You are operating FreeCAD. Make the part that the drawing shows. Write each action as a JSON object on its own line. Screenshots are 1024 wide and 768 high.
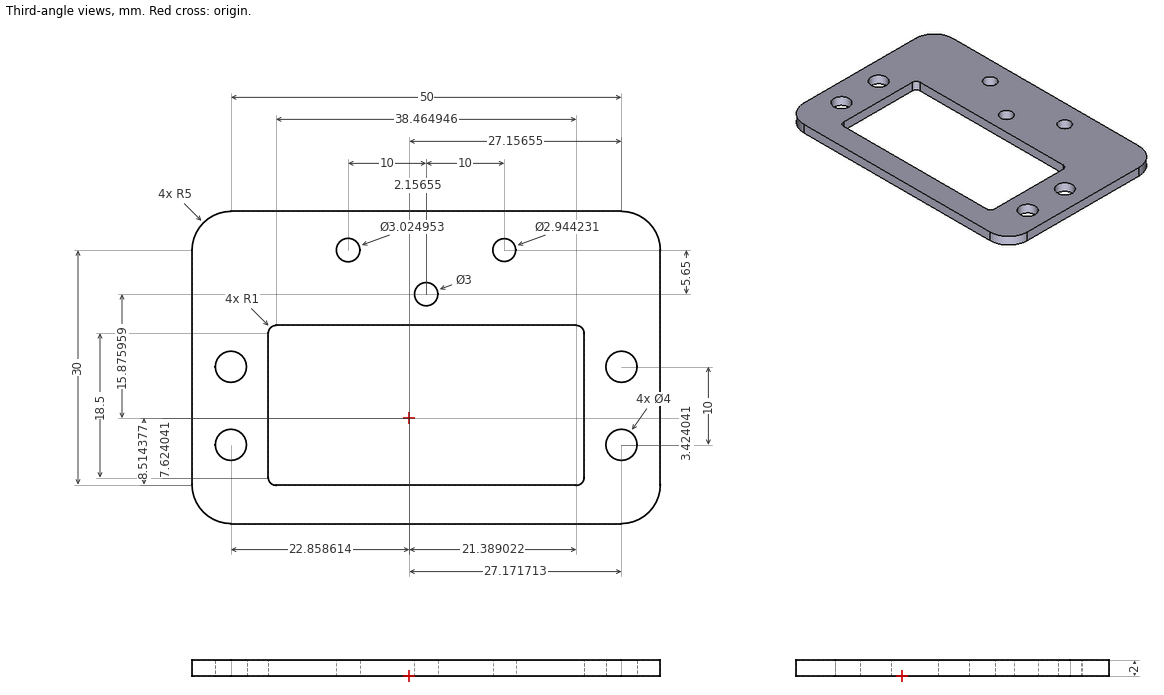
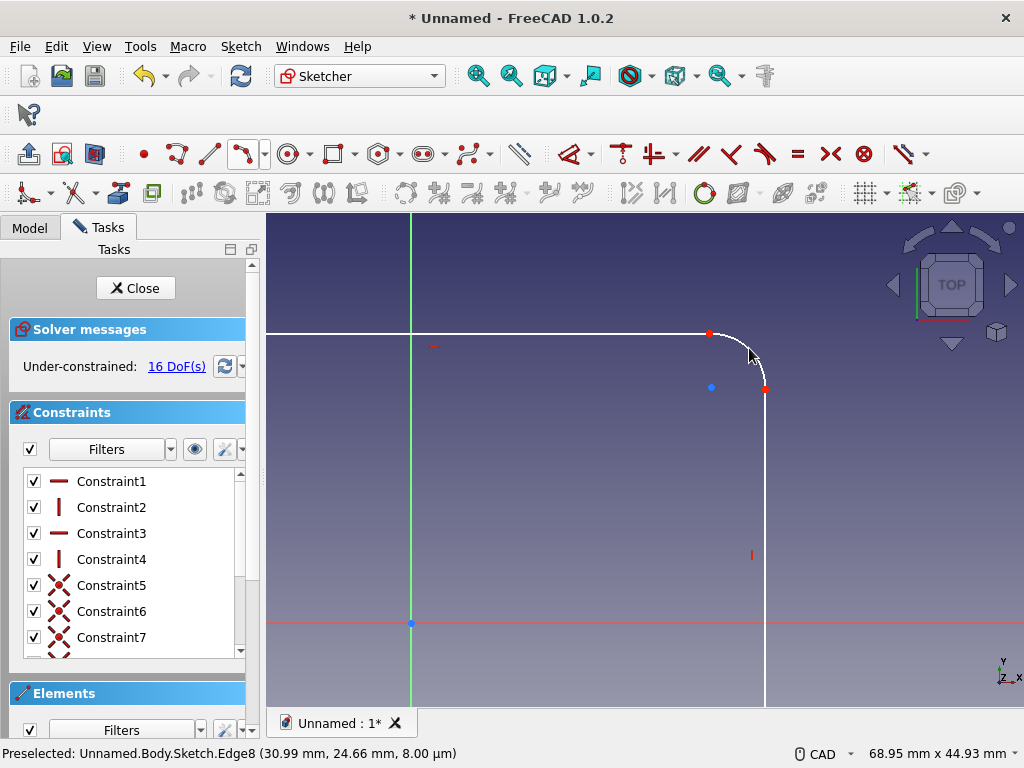
{"action": "left_click", "coordinate": [545, 334]}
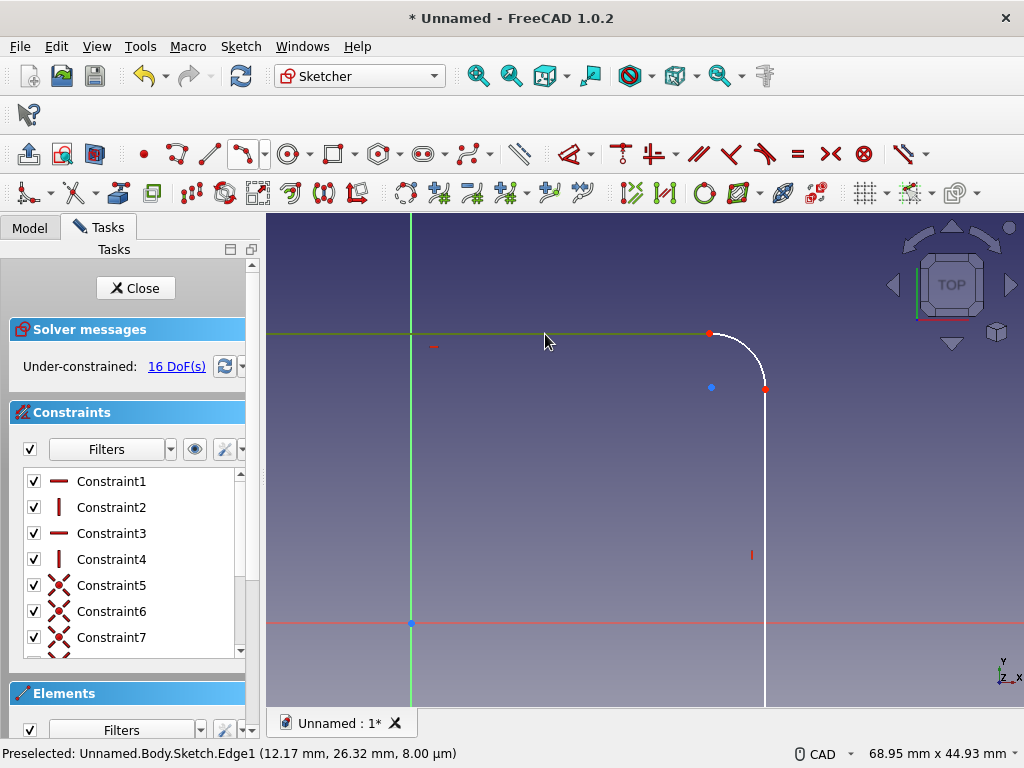
{"action": "scroll", "coordinate": [749, 348], "scroll_direction": "down", "scroll_amount": 3}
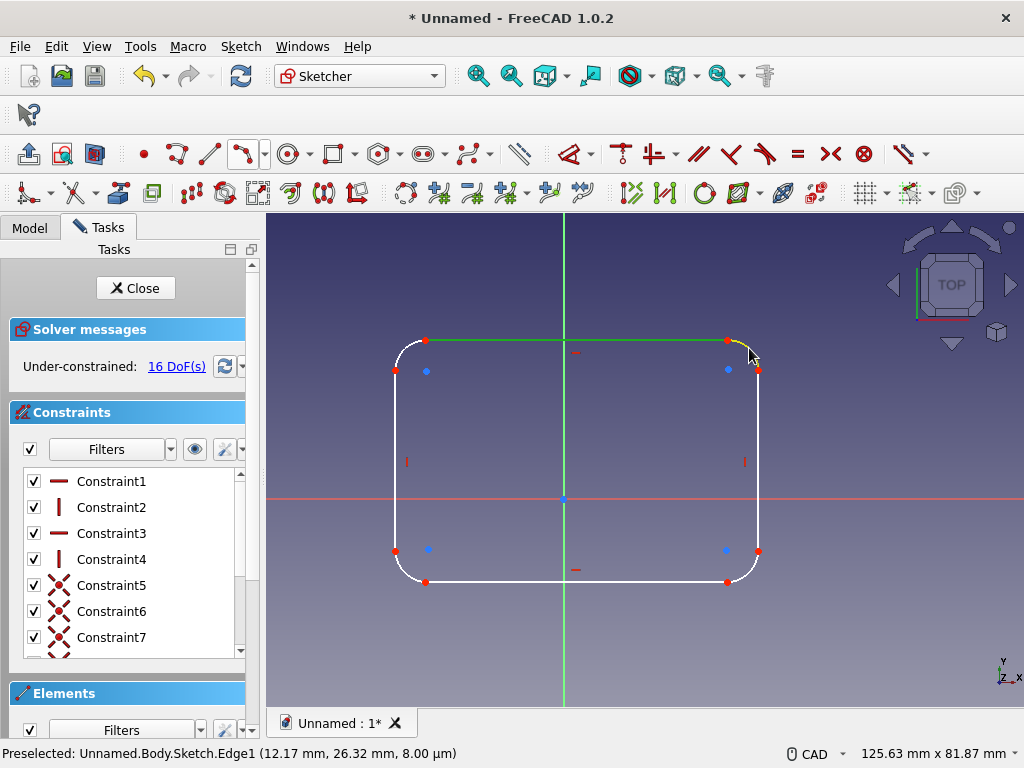
{"action": "left_click", "coordinate": [412, 344]}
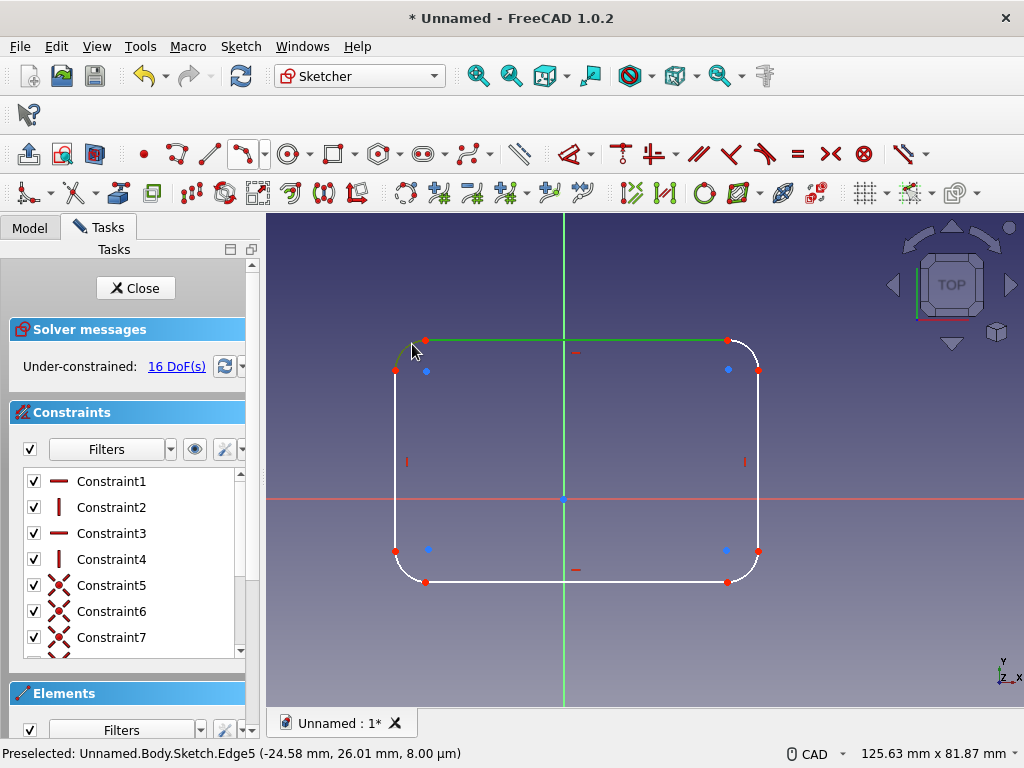
{"action": "left_click", "coordinate": [765, 154]}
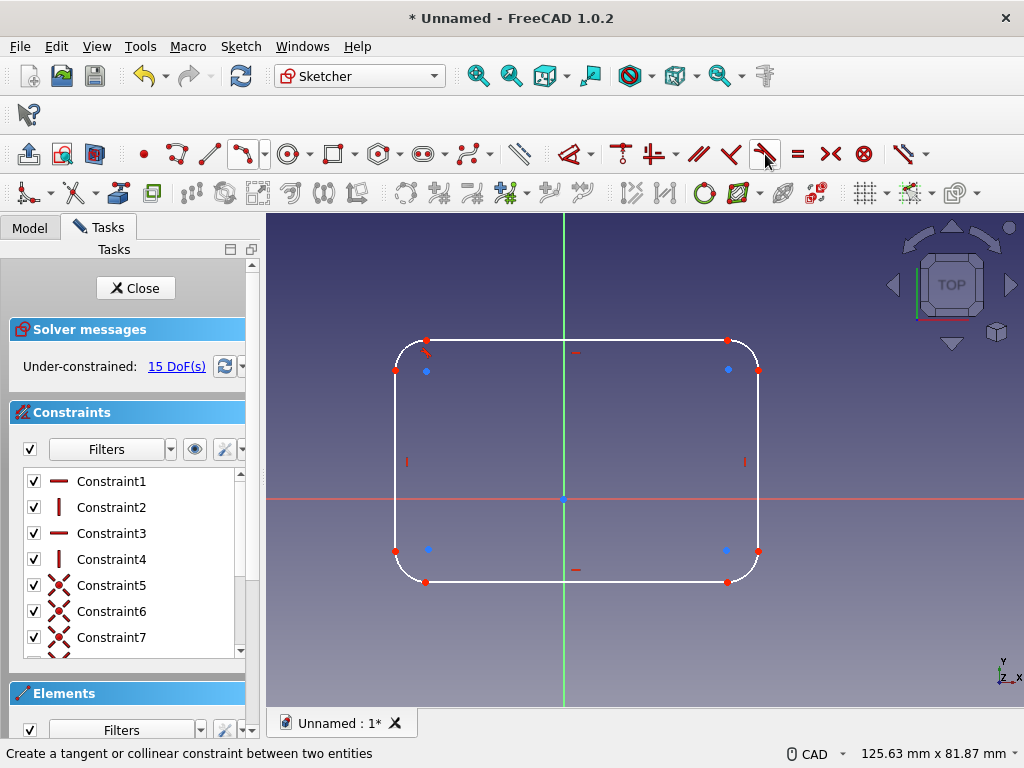
{"action": "left_click", "coordinate": [637, 340]}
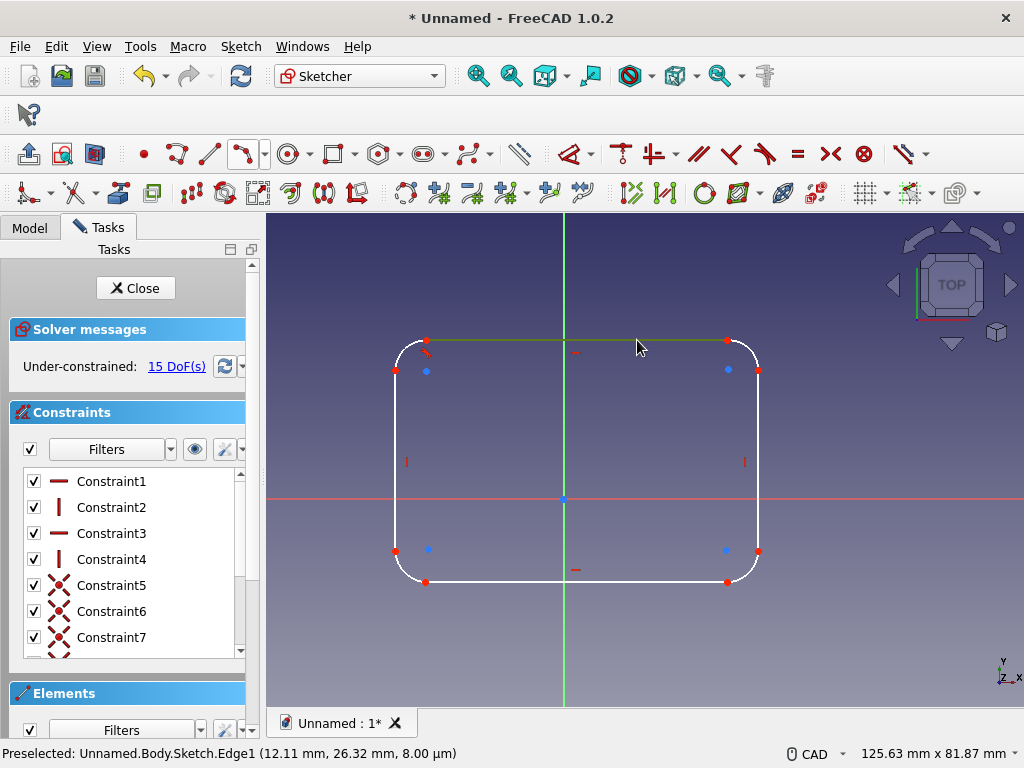
{"action": "left_click", "coordinate": [755, 357]}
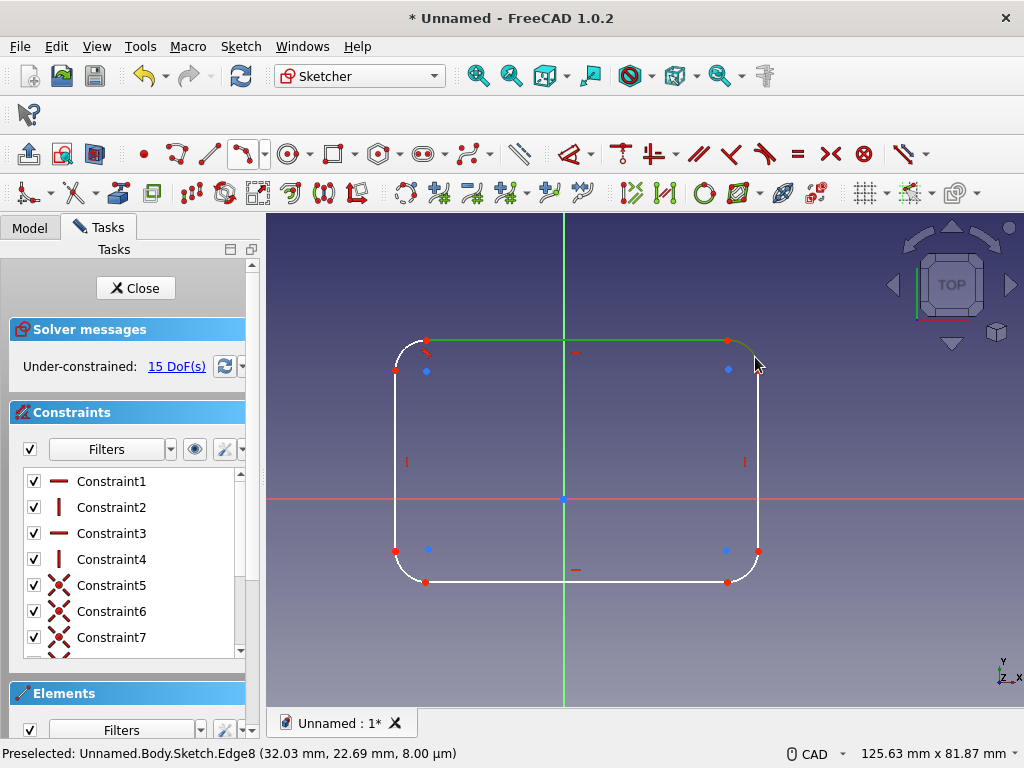
{"action": "left_click", "coordinate": [765, 154]}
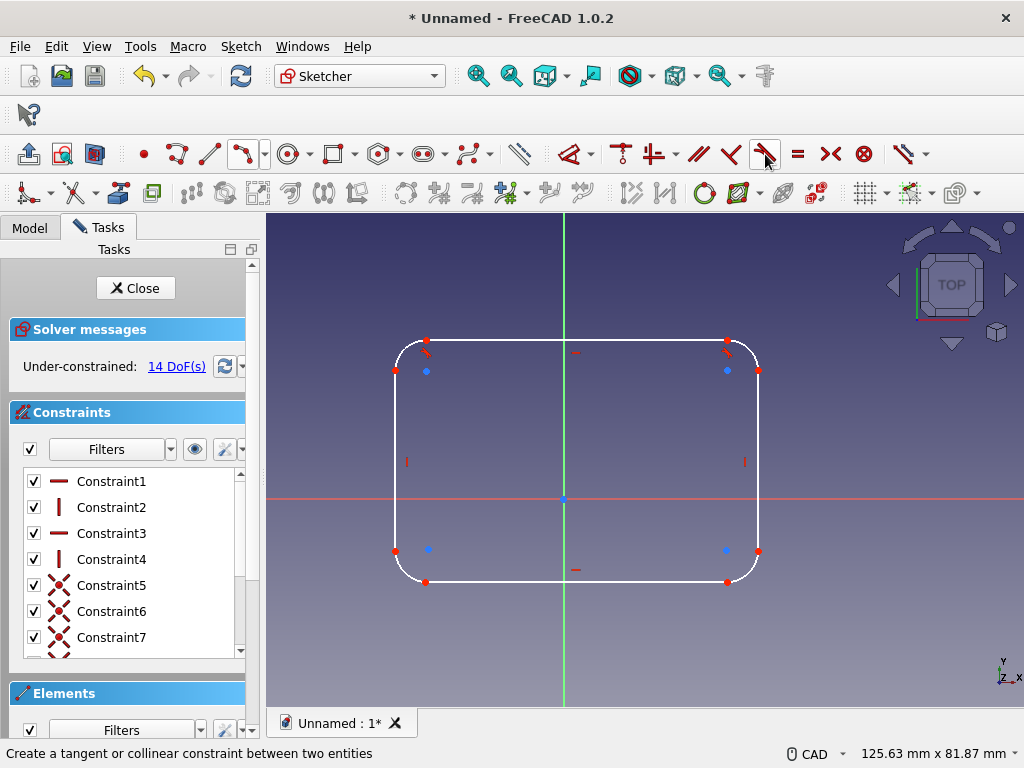
{"action": "left_click", "coordinate": [395, 425]}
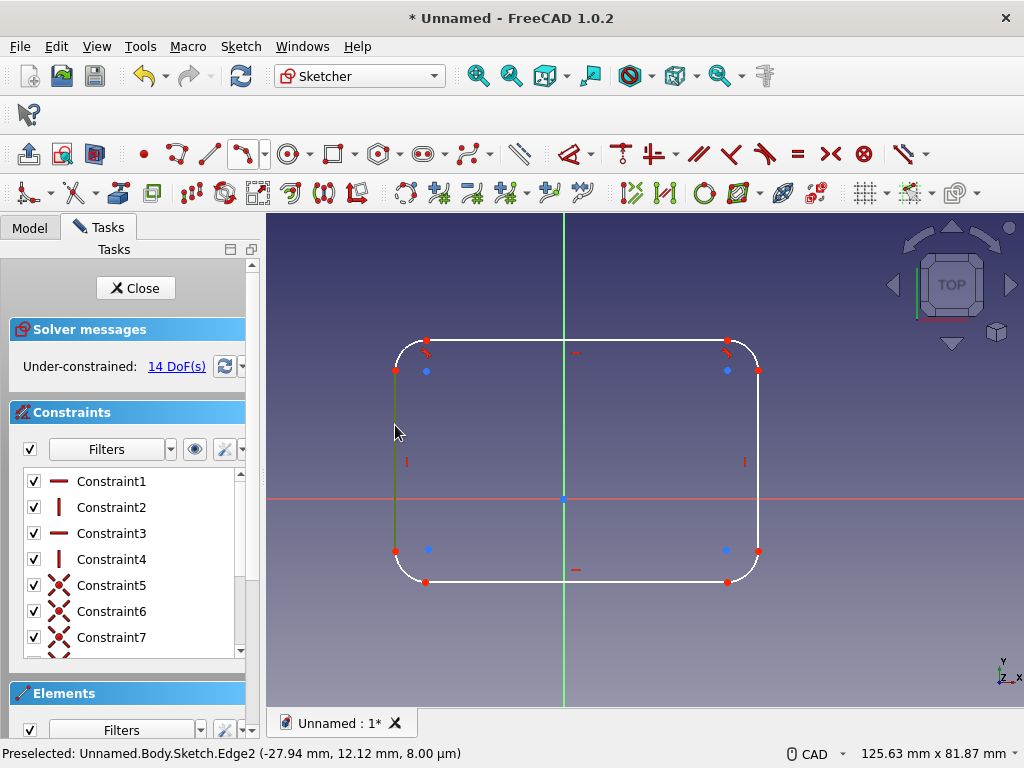
{"action": "left_click", "coordinate": [412, 344]}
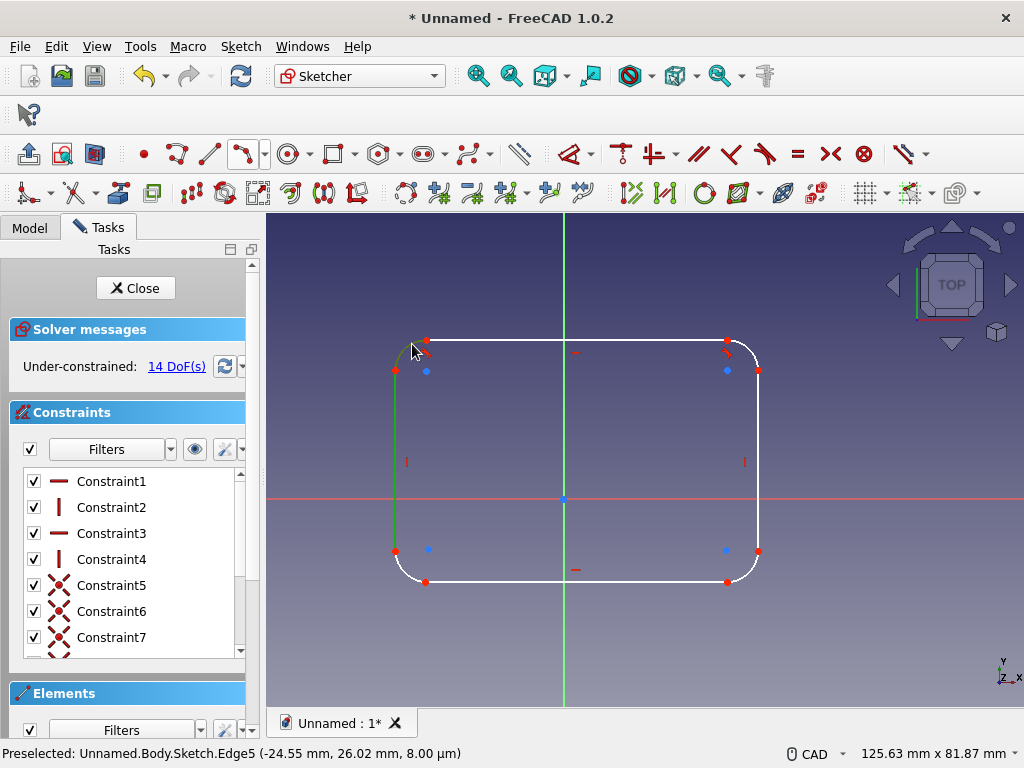
{"action": "key", "text": "t"}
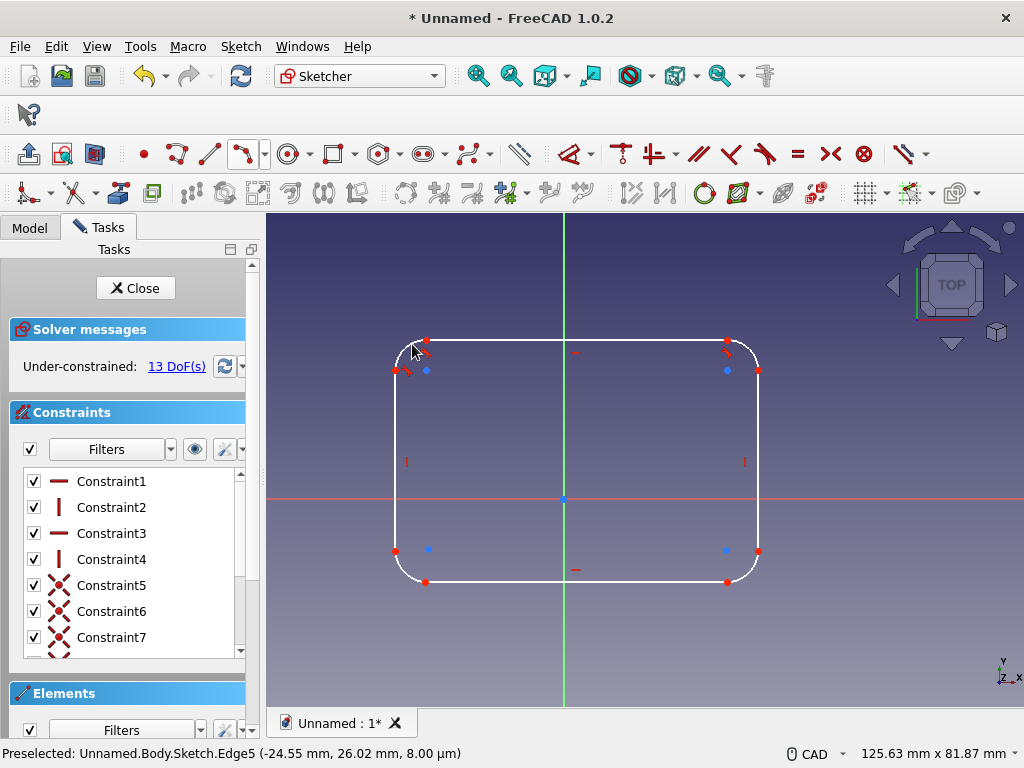
{"action": "left_click", "coordinate": [395, 425]}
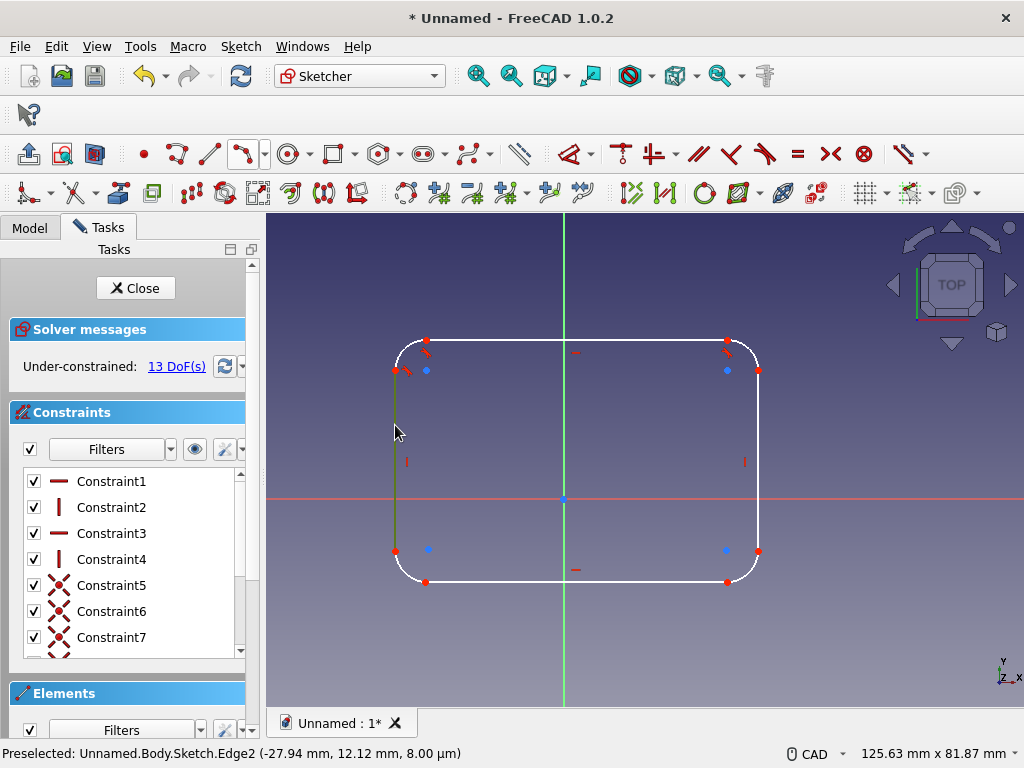
{"action": "left_click", "coordinate": [399, 565]}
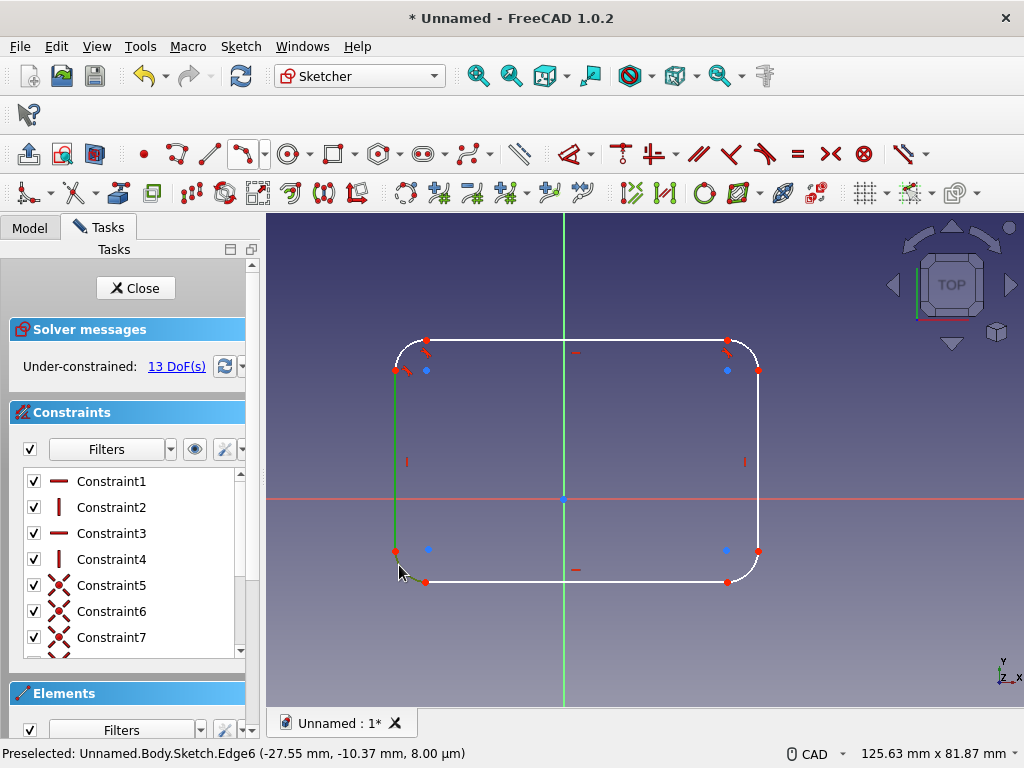
{"action": "left_click", "coordinate": [765, 154]}